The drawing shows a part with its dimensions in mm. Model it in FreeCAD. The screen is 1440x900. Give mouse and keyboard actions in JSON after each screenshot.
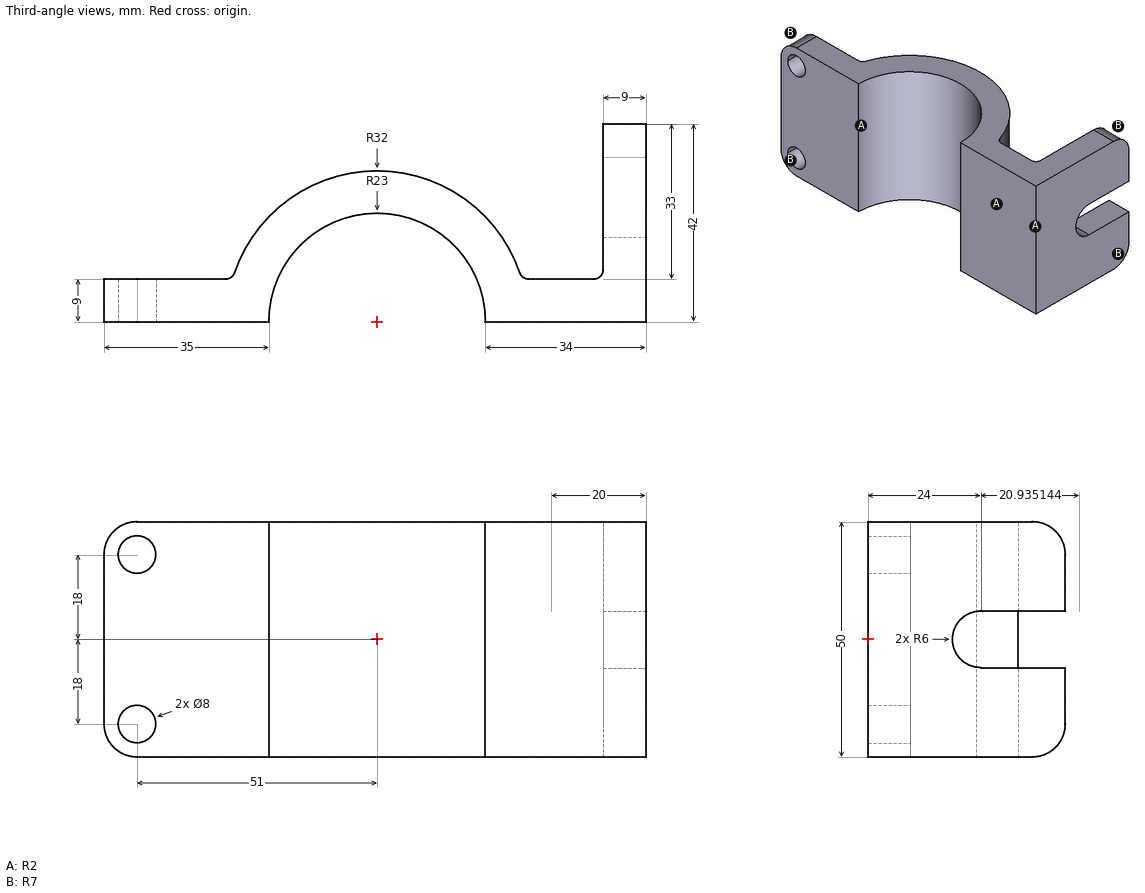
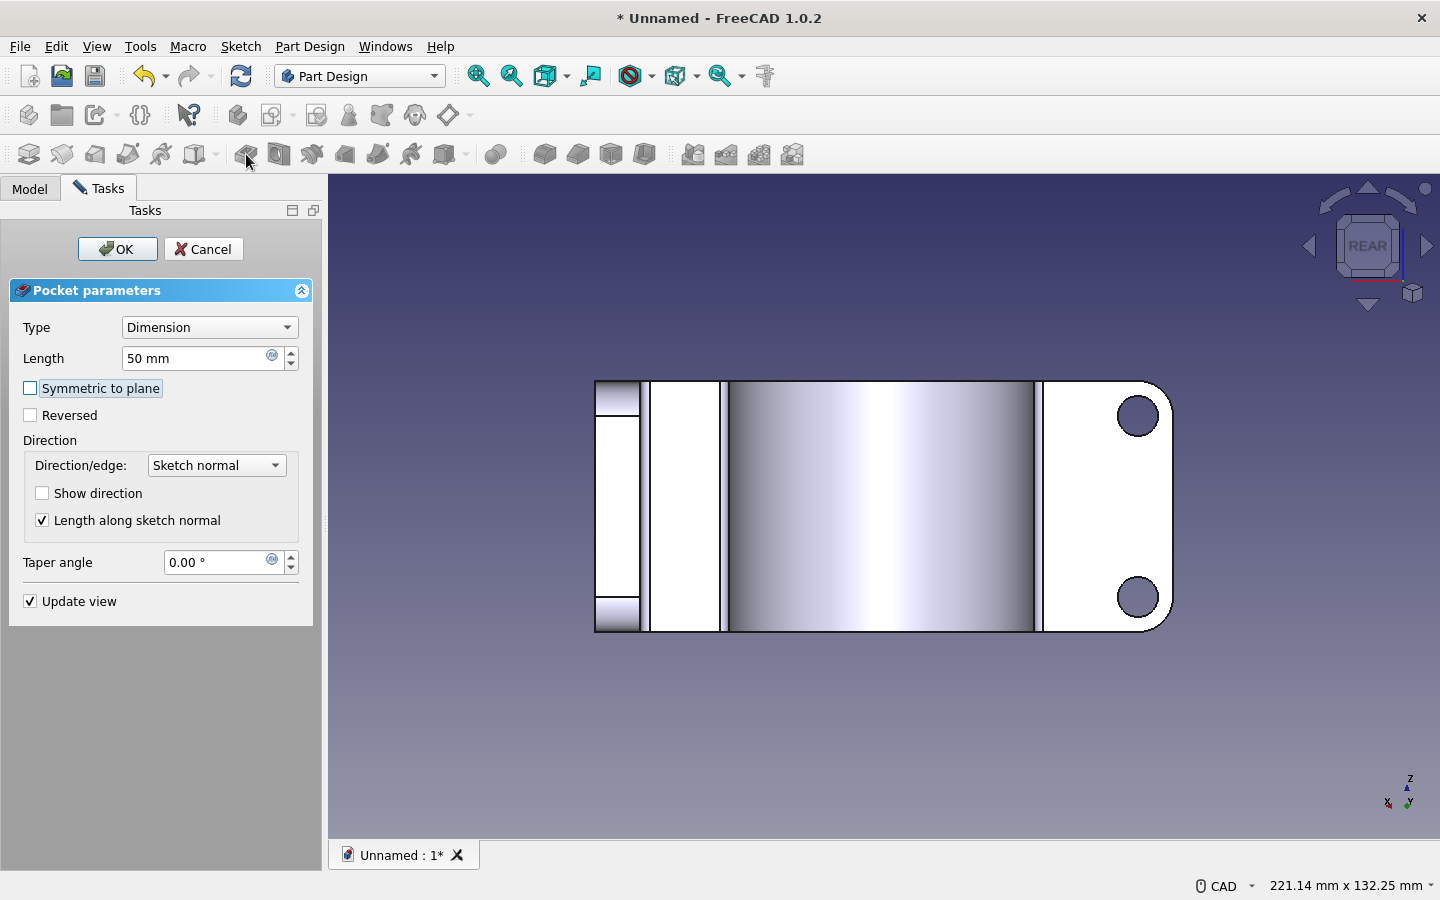
{"action": "left_click", "coordinate": [118, 249]}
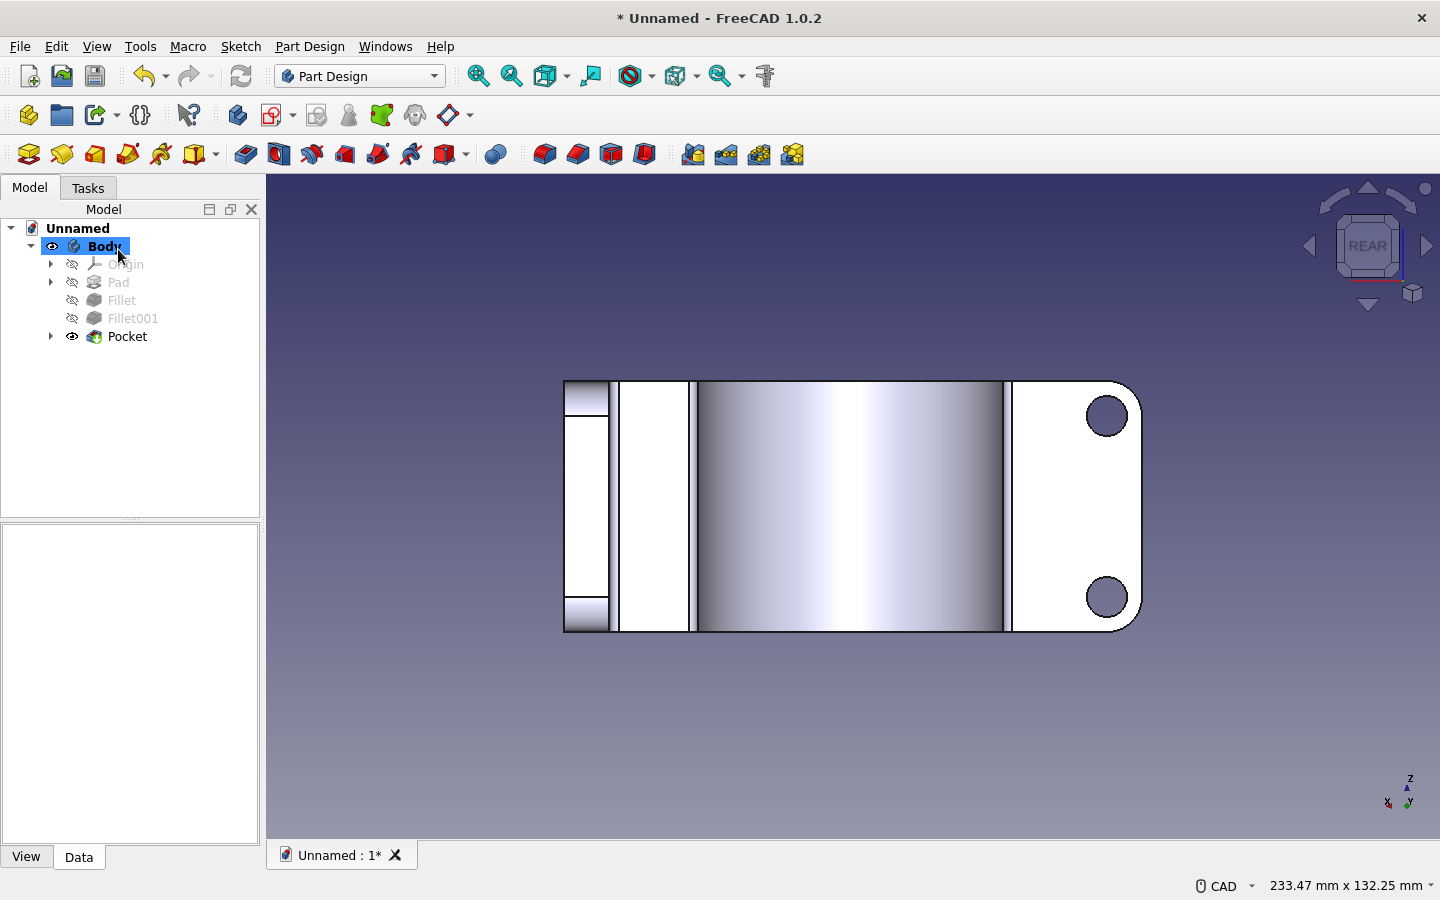
{"action": "key", "text": "0"}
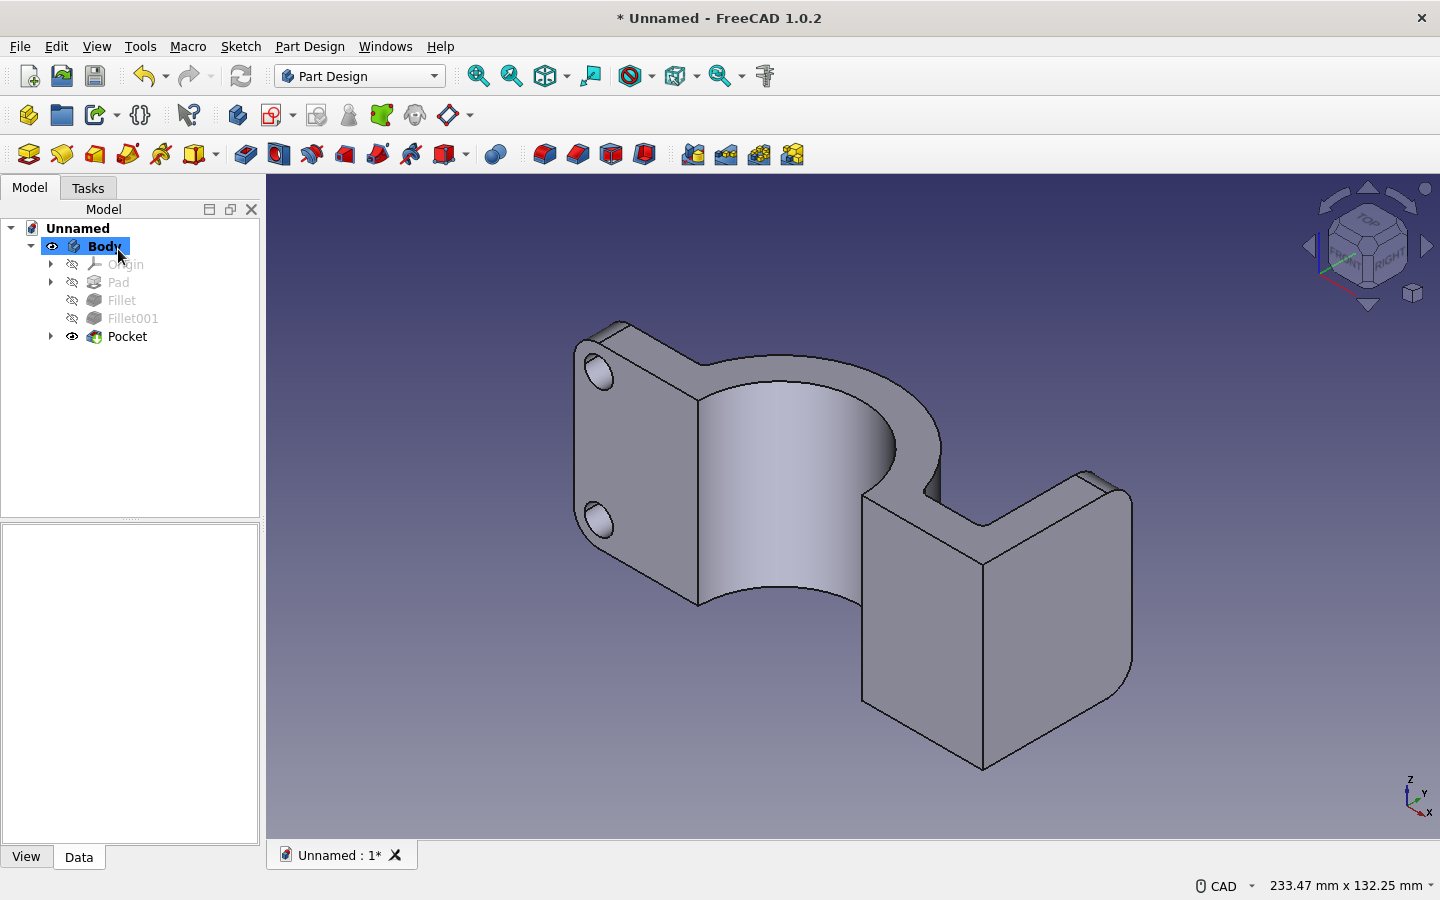
{"action": "left_click", "coordinate": [1057, 624]}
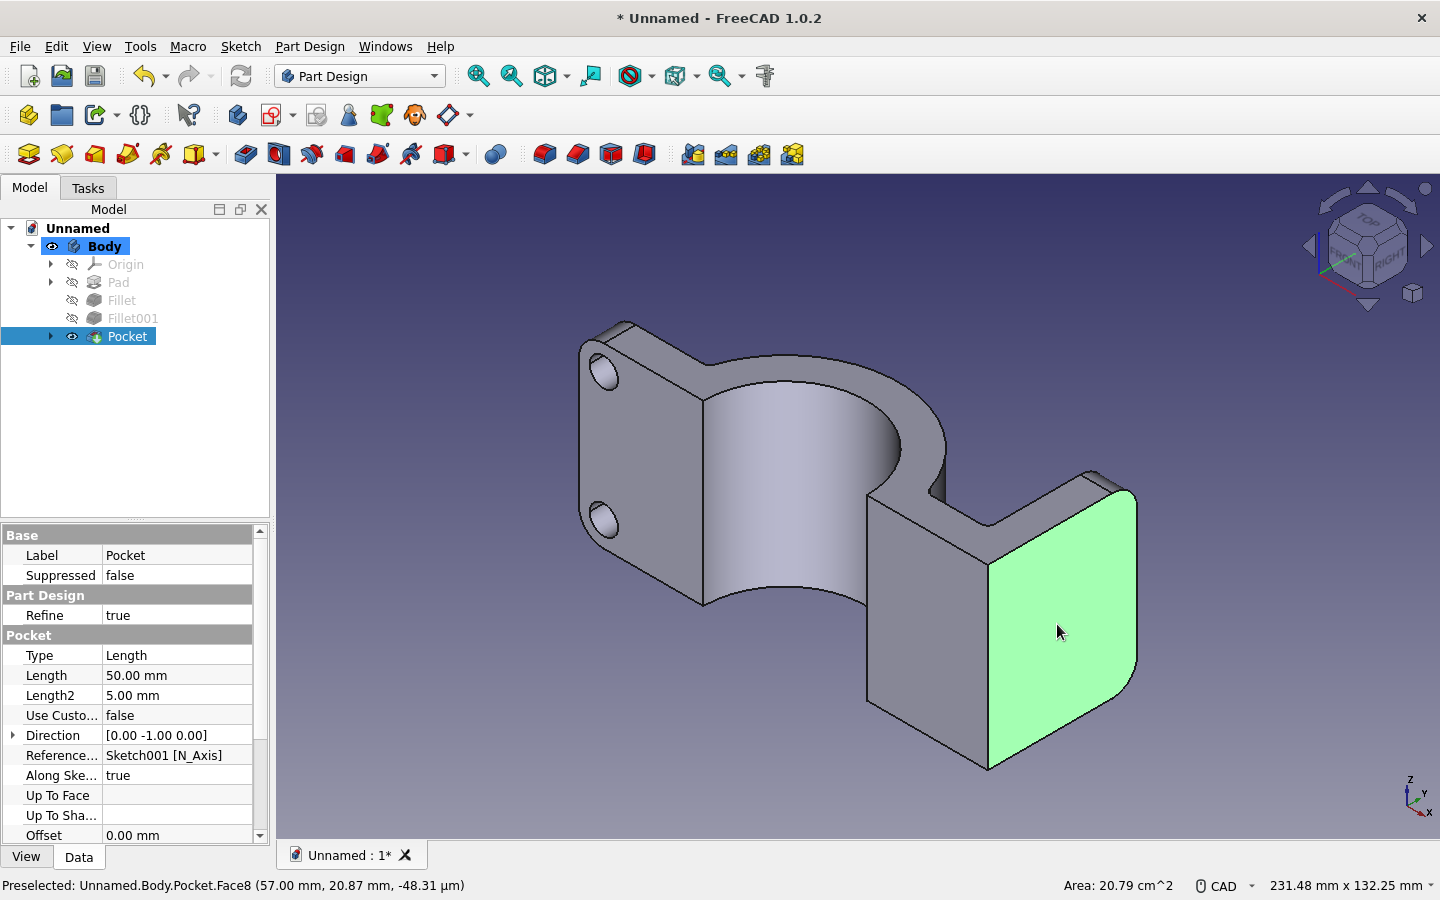
{"action": "left_click", "coordinate": [270, 116]}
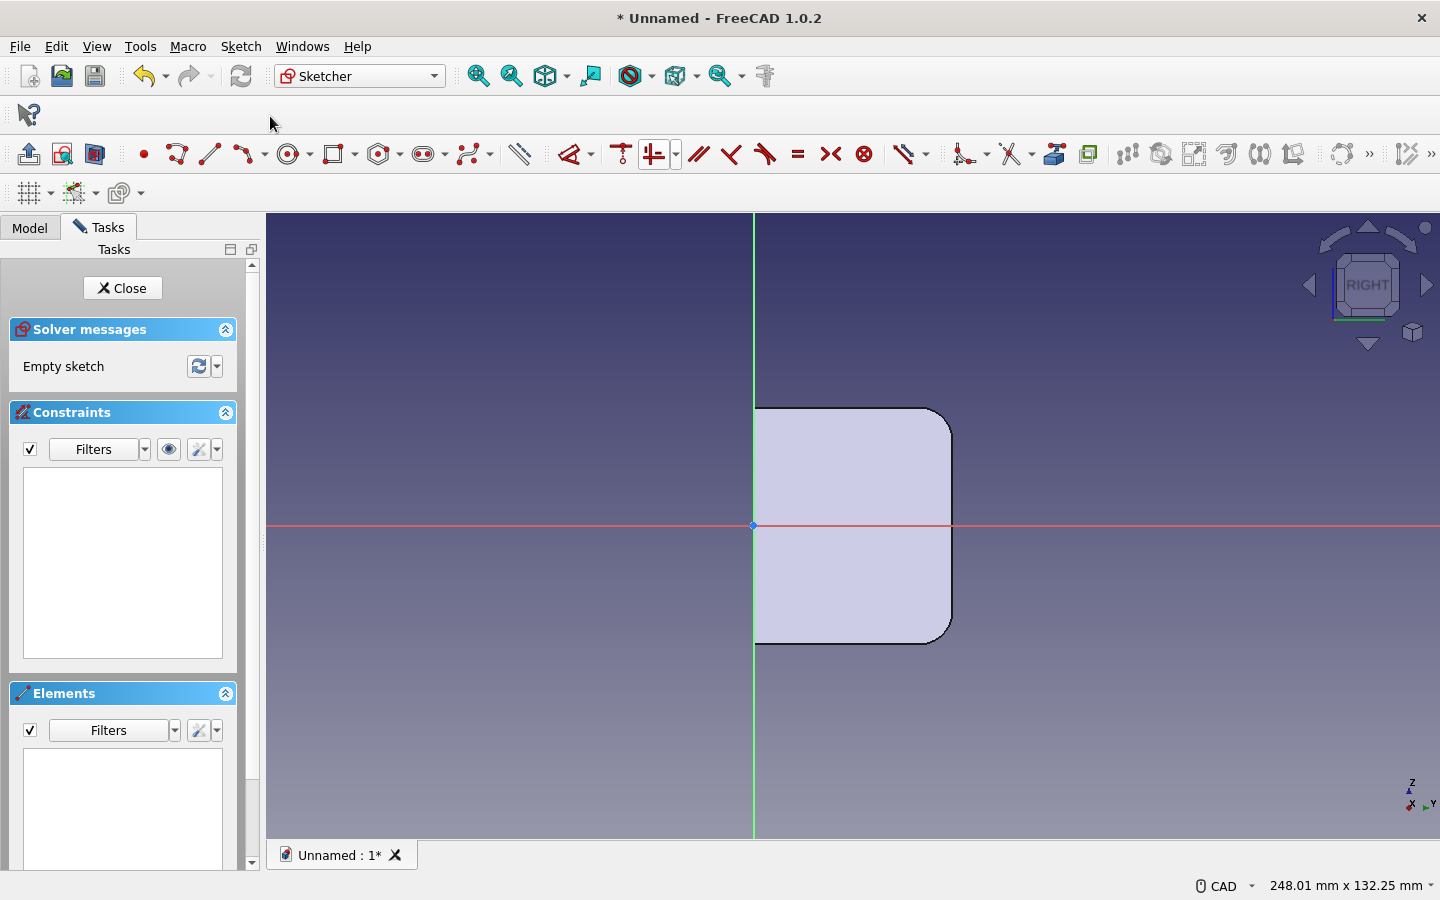
{"action": "scroll", "coordinate": [926, 526], "scroll_direction": "up", "scroll_amount": 5}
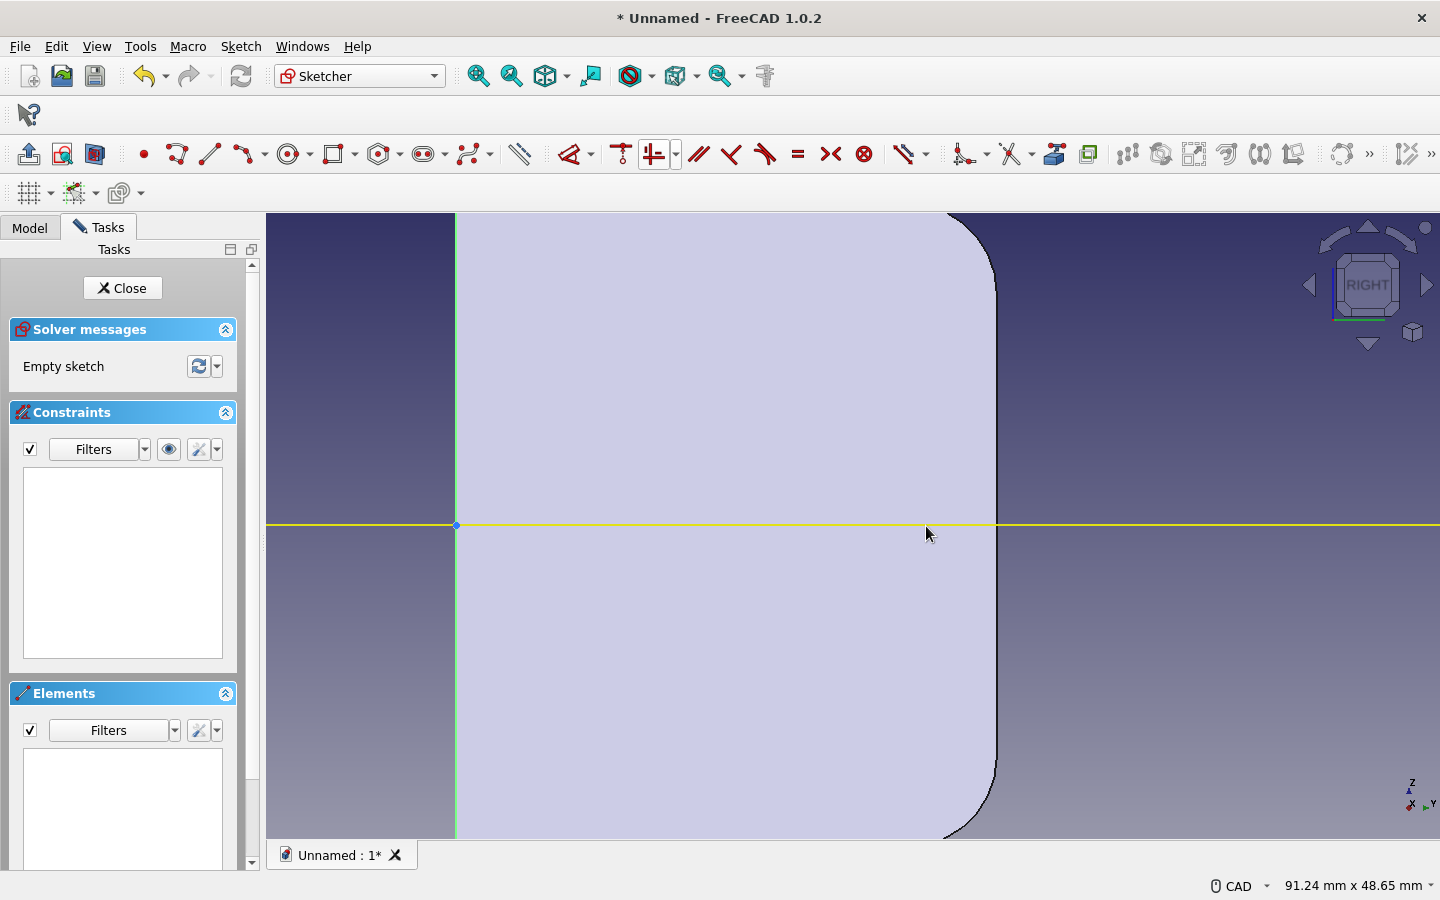
{"action": "left_click", "coordinate": [422, 154]}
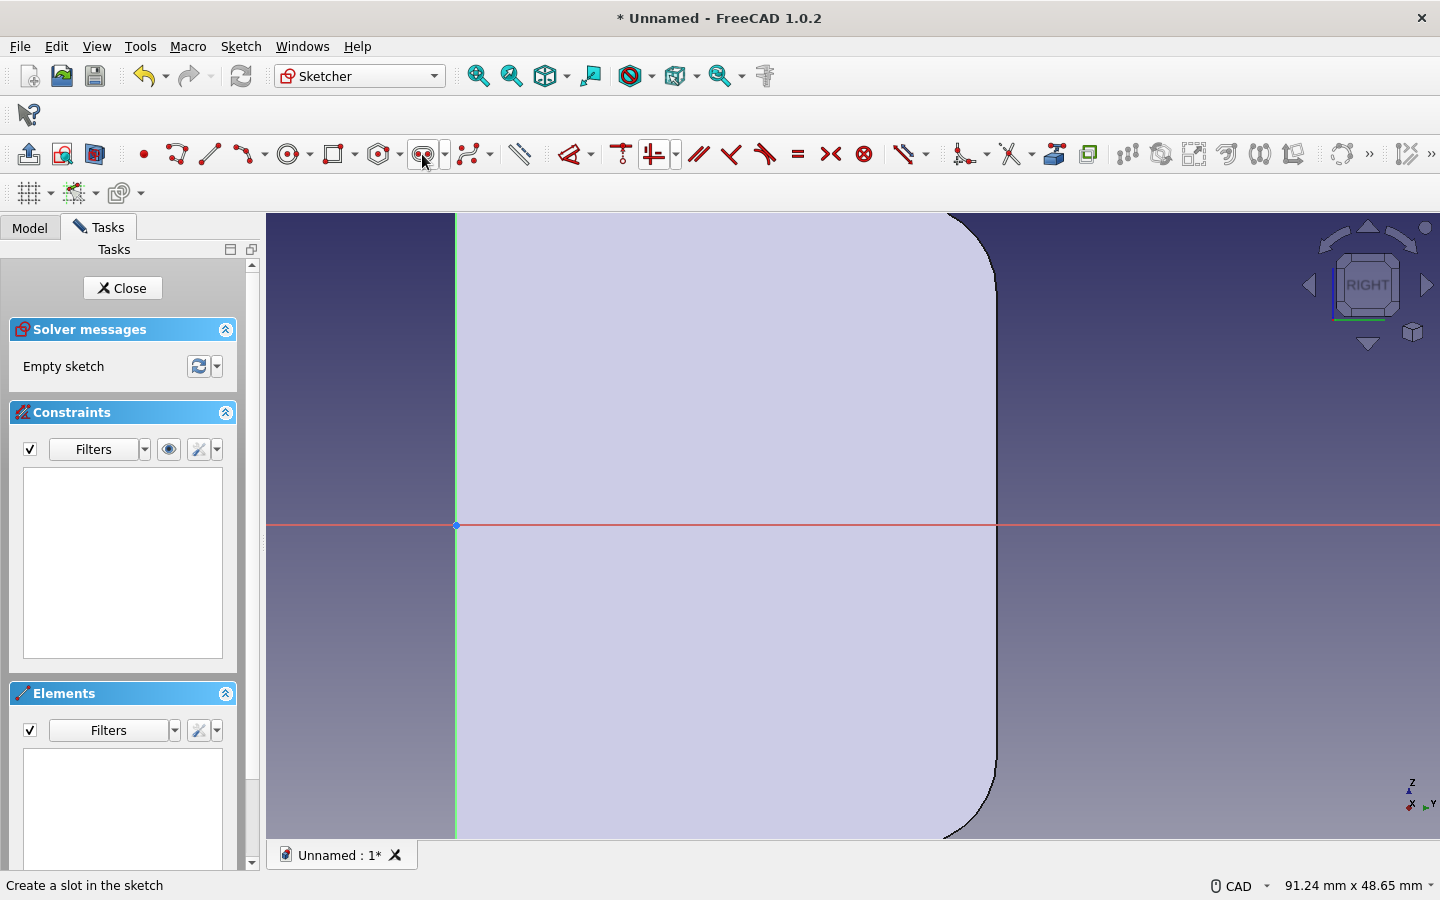
{"action": "left_click", "coordinate": [765, 525]}